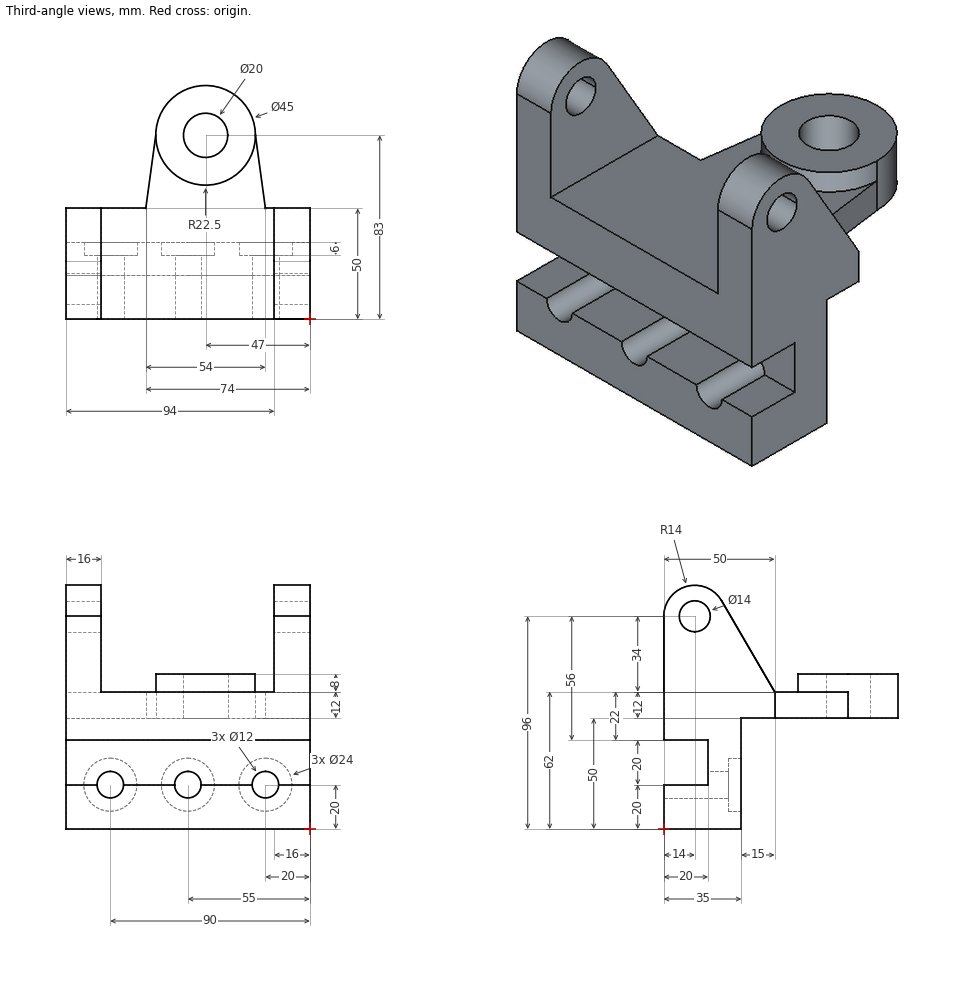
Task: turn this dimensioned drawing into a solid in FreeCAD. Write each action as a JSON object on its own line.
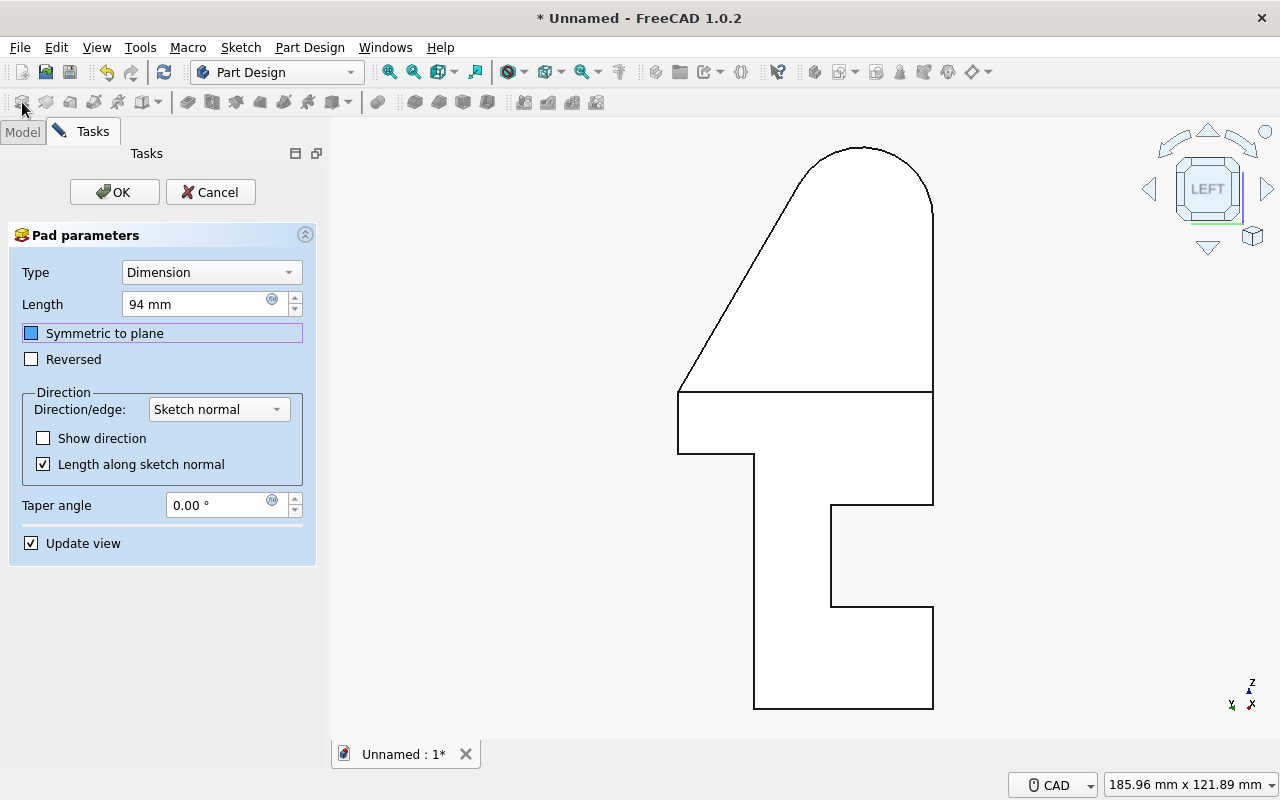
{"action": "left_click", "coordinate": [115, 192]}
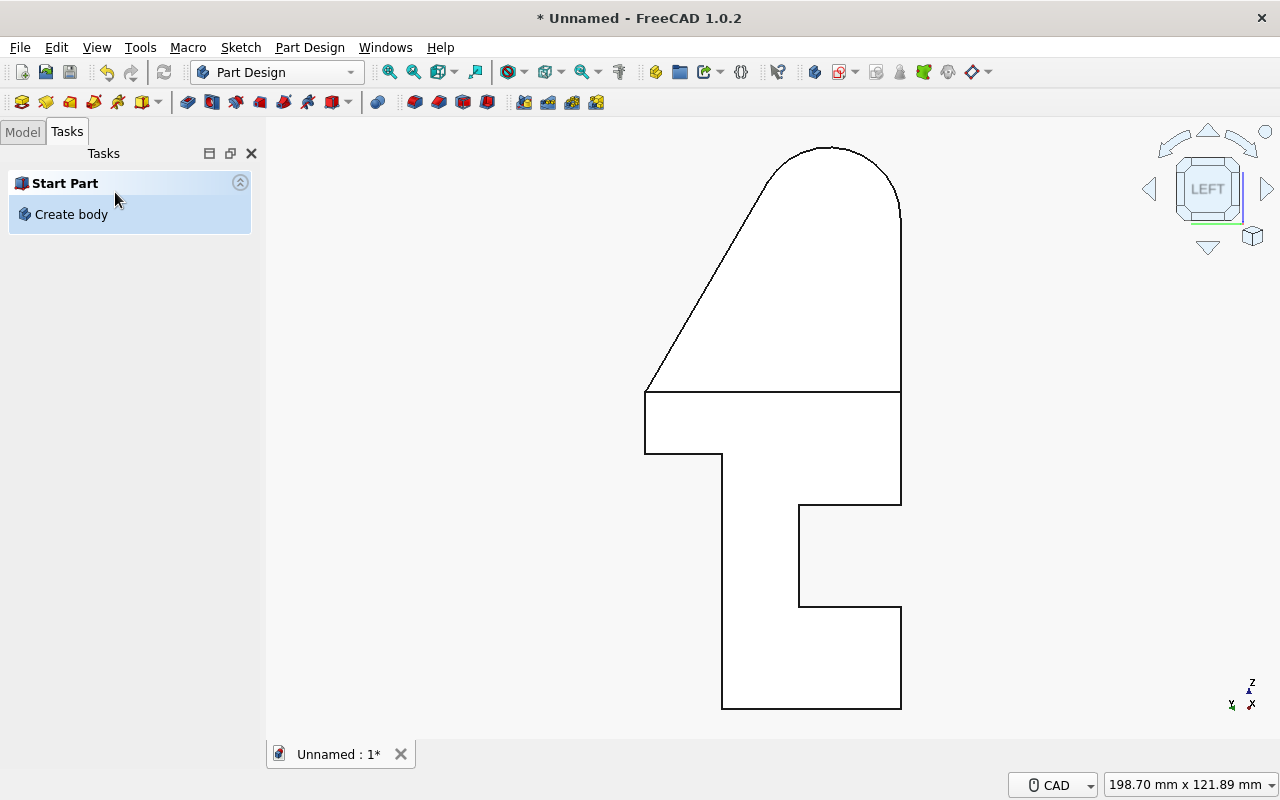
{"action": "left_click", "coordinate": [23, 131]}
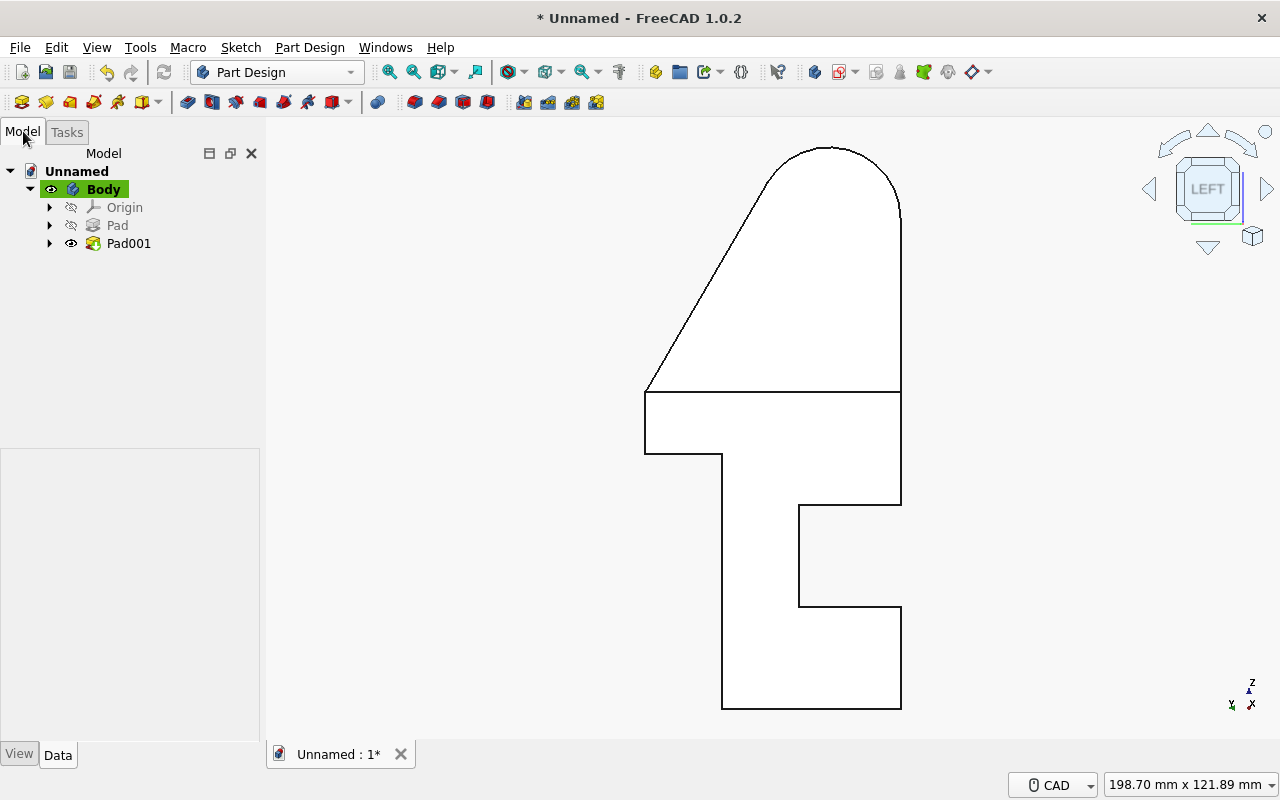
{"action": "left_click", "coordinate": [50, 207]}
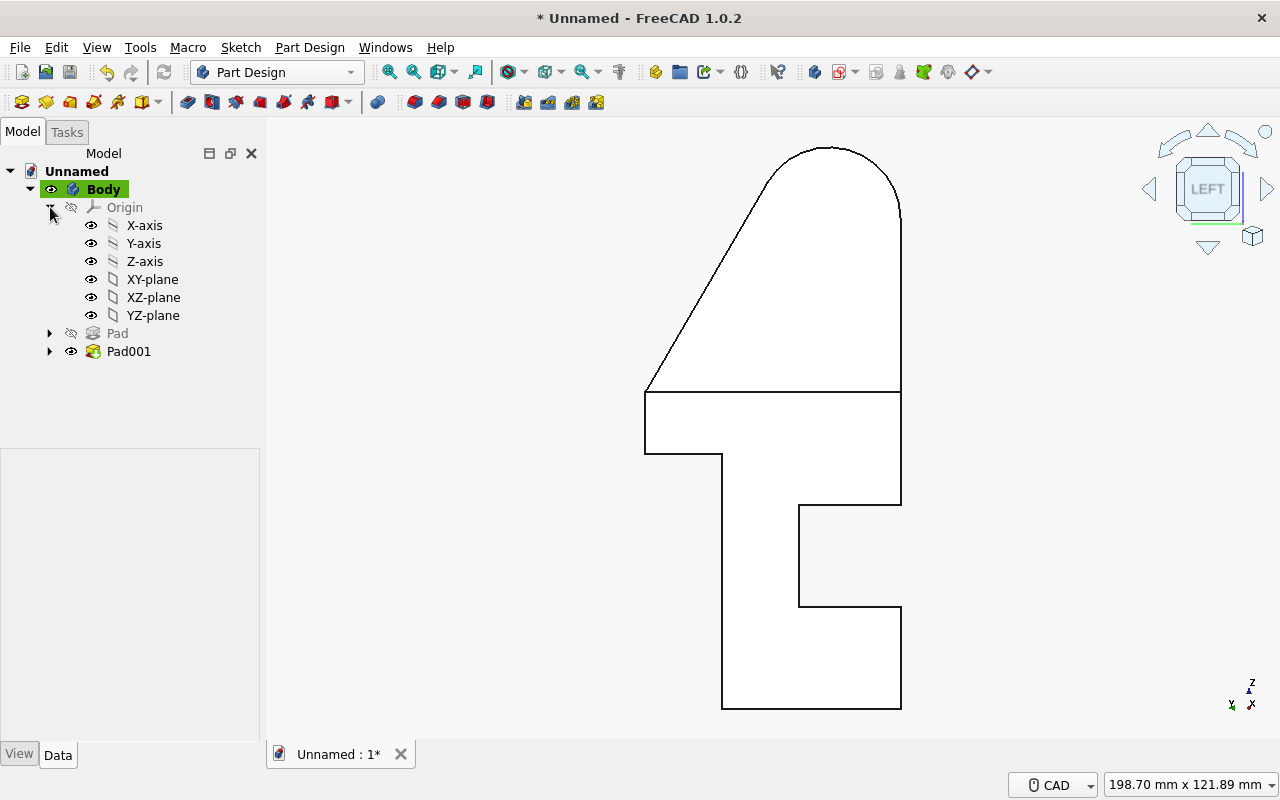
{"action": "left_click", "coordinate": [136, 315]}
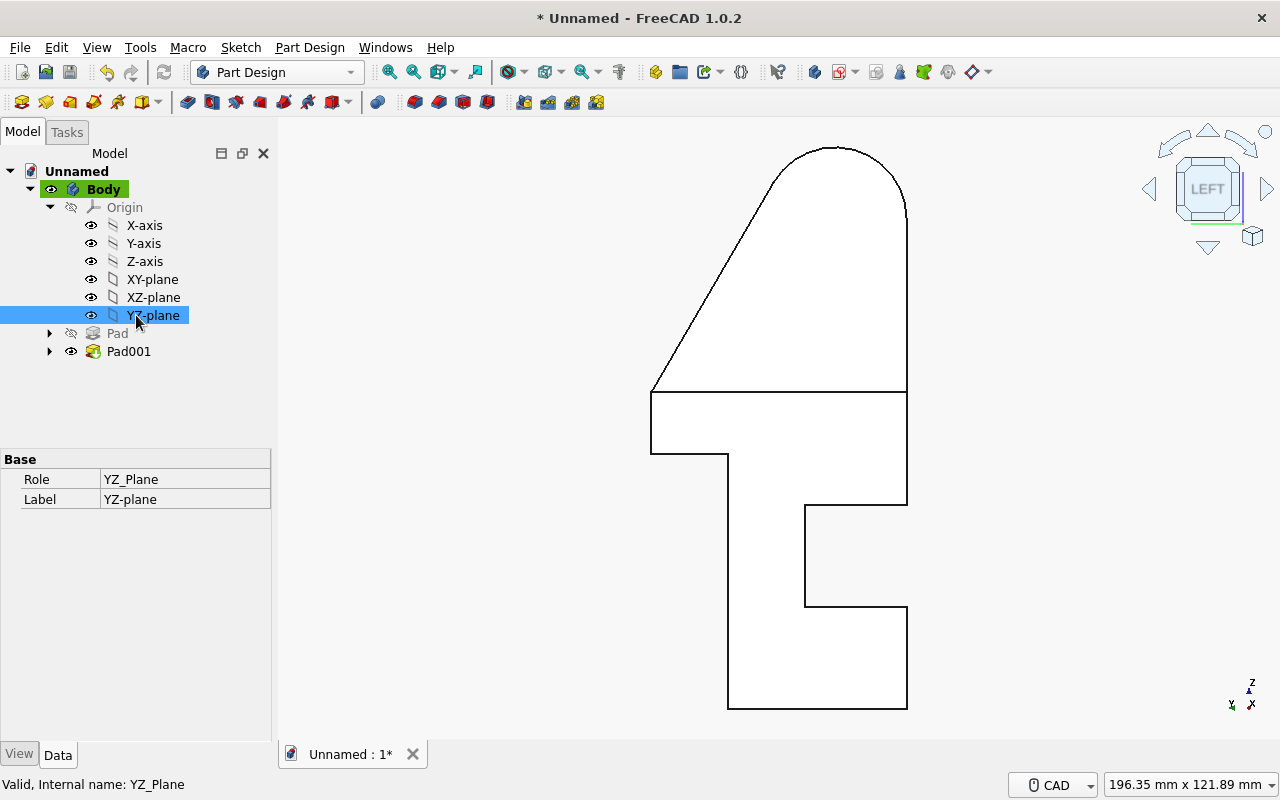
{"action": "left_click", "coordinate": [972, 72]}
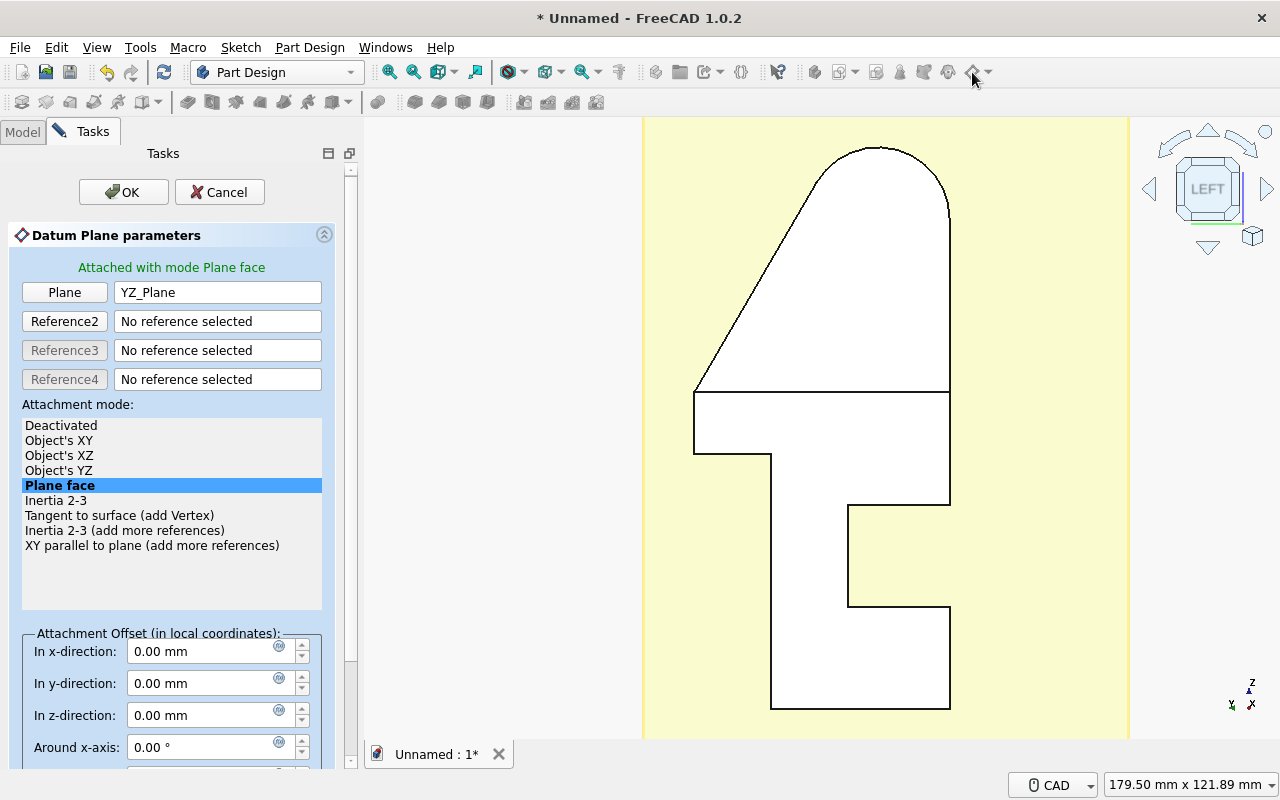
{"action": "triple_click", "coordinate": [210, 715]}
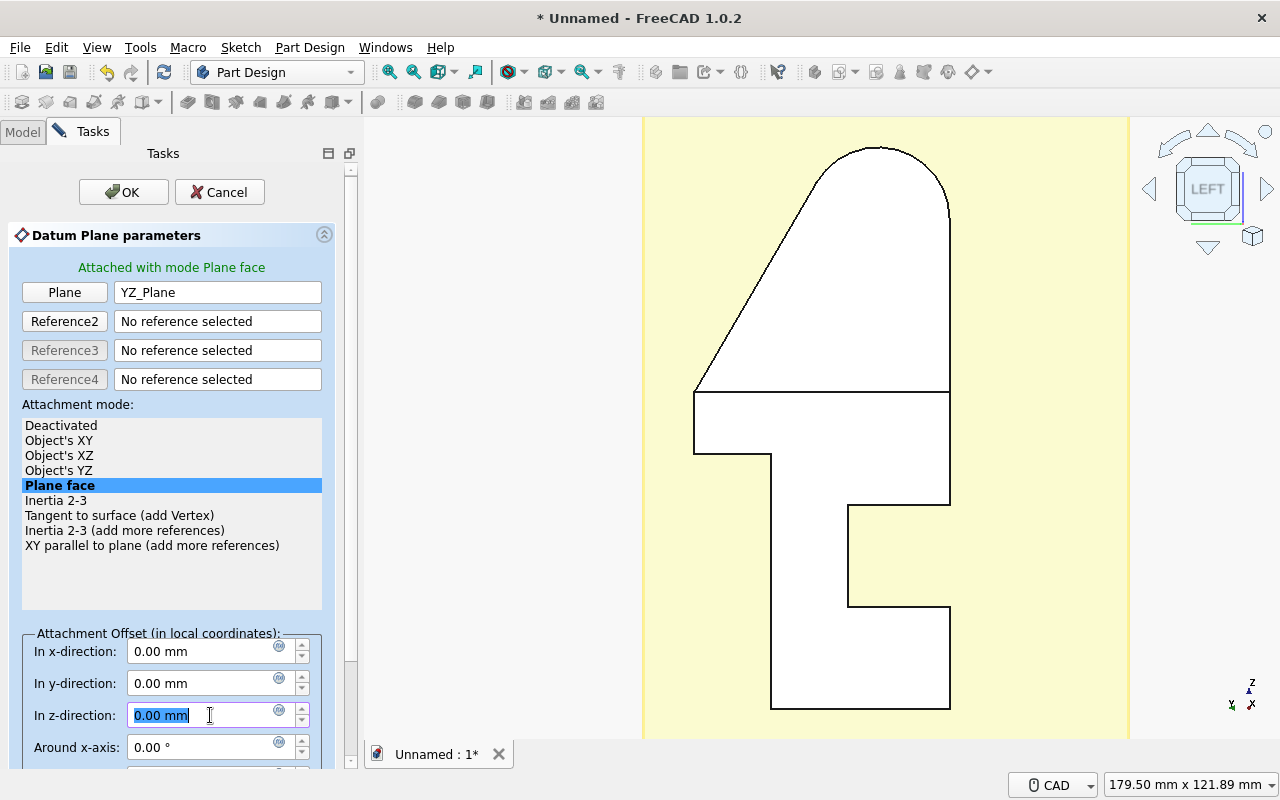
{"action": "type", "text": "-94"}
{"action": "key", "text": "Tab"}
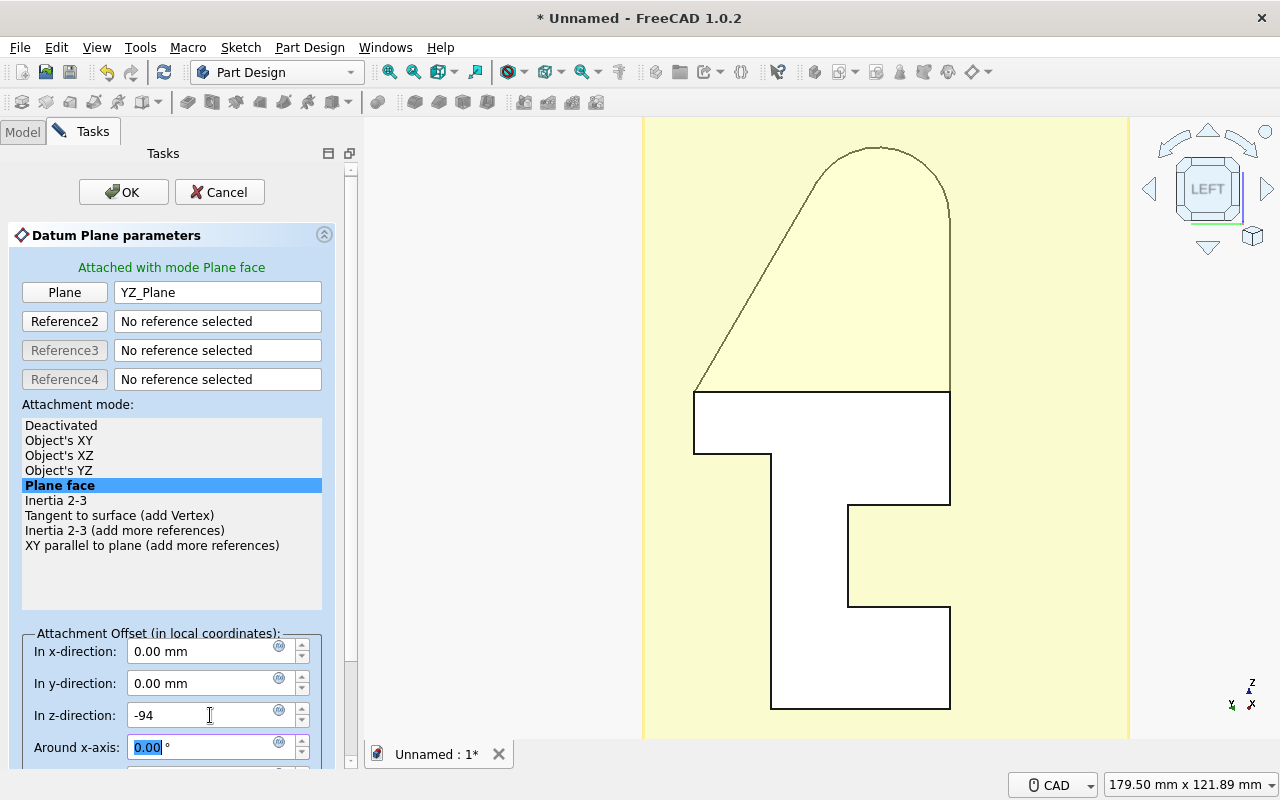
{"action": "left_click", "coordinate": [124, 192]}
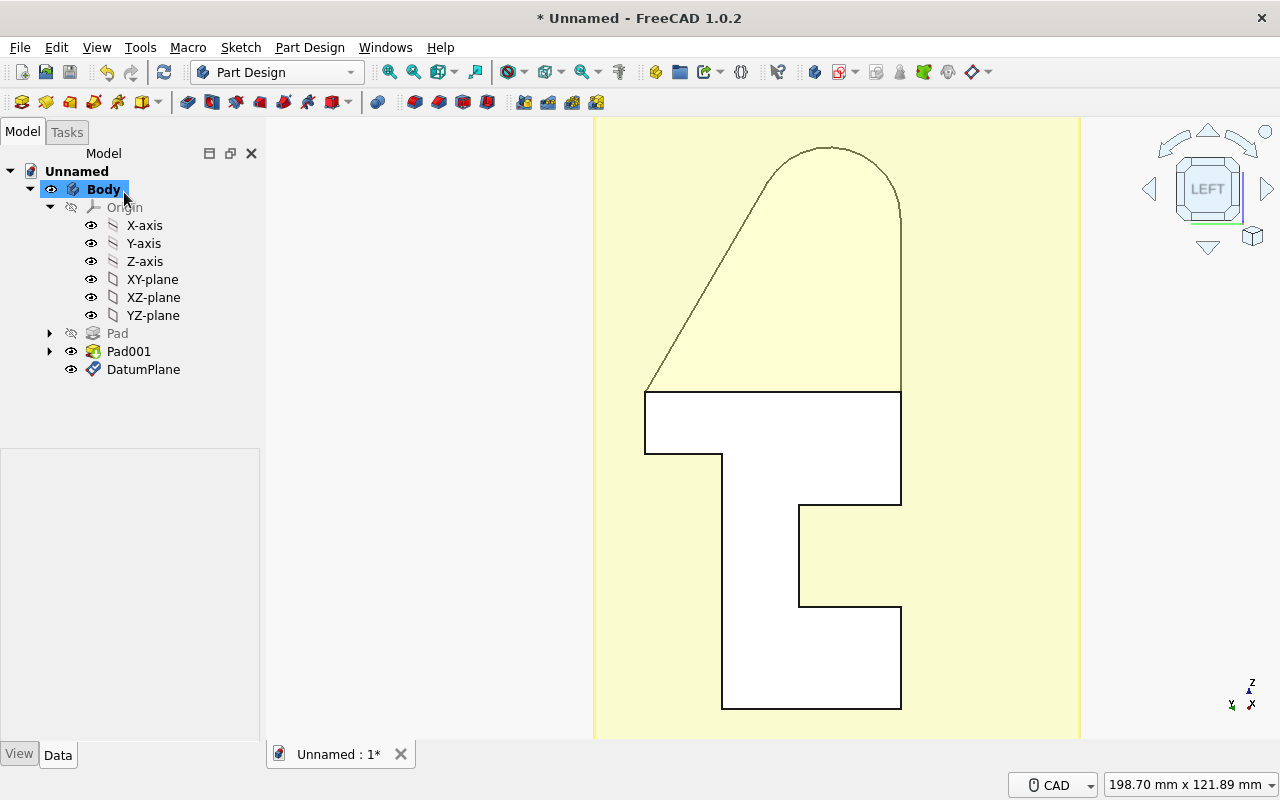
{"action": "left_click", "coordinate": [116, 369]}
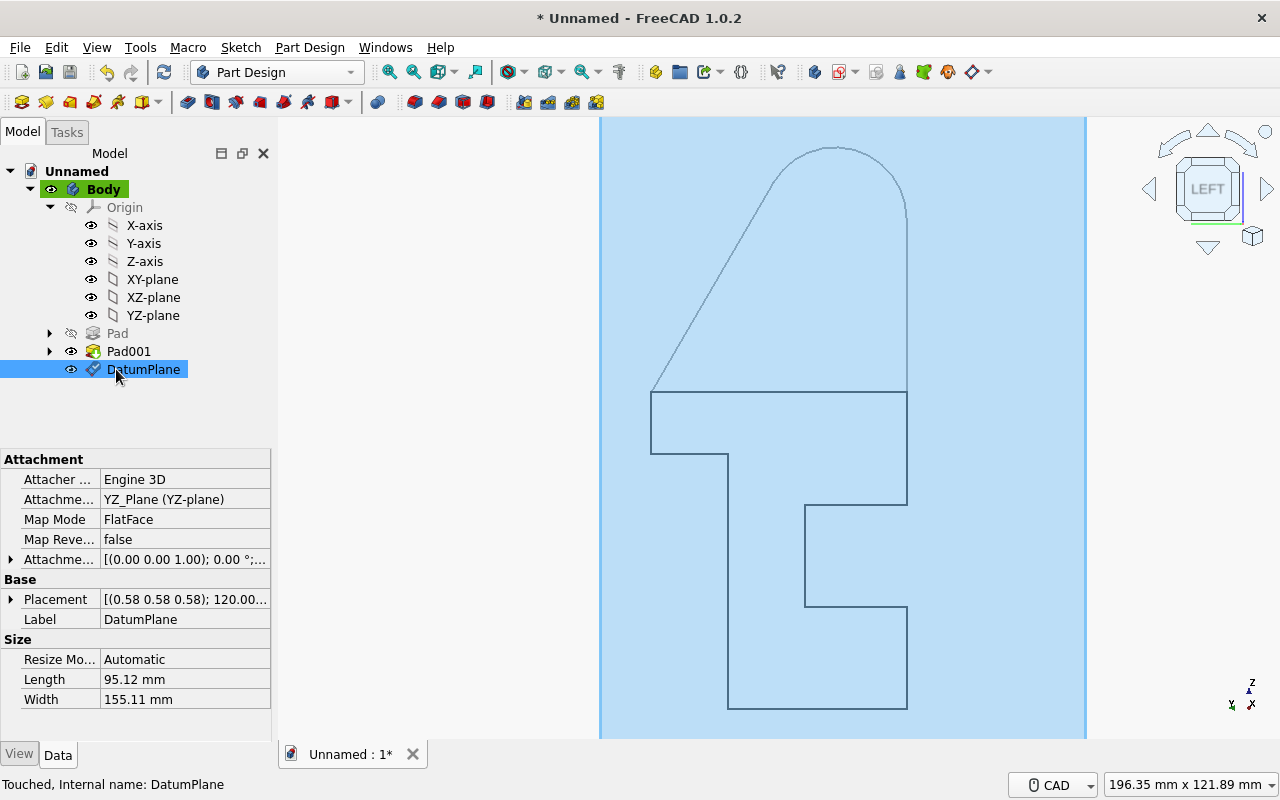
{"action": "left_click", "coordinate": [840, 72]}